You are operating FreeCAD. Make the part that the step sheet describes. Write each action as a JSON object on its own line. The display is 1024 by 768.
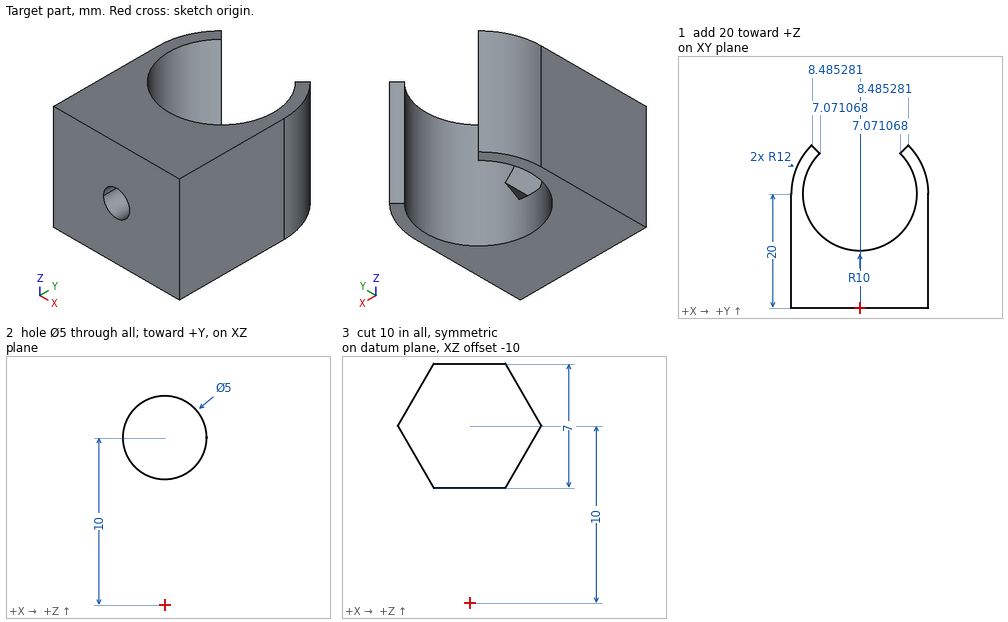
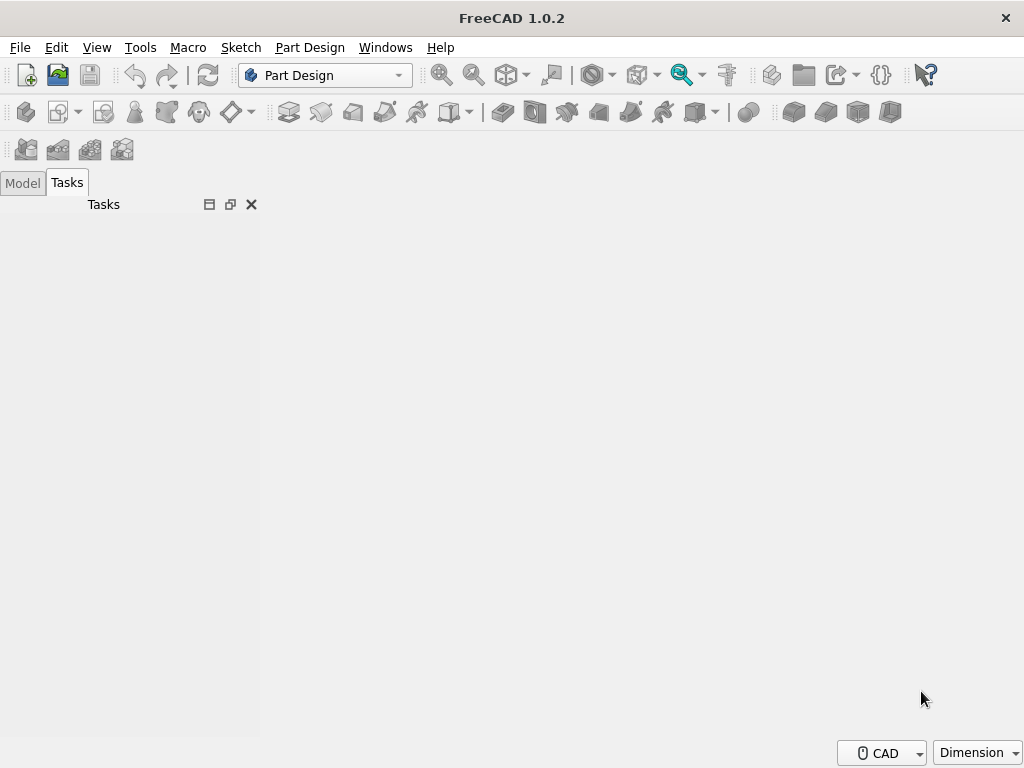
{"action": "left_click", "coordinate": [26, 76]}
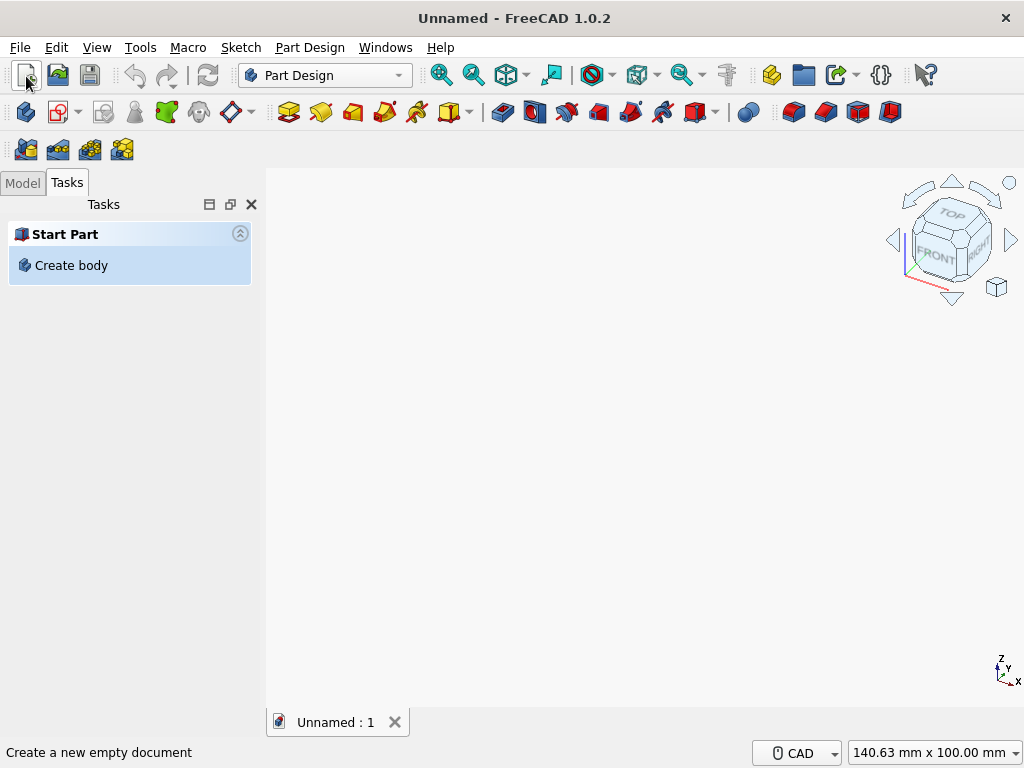
{"action": "left_click", "coordinate": [58, 112]}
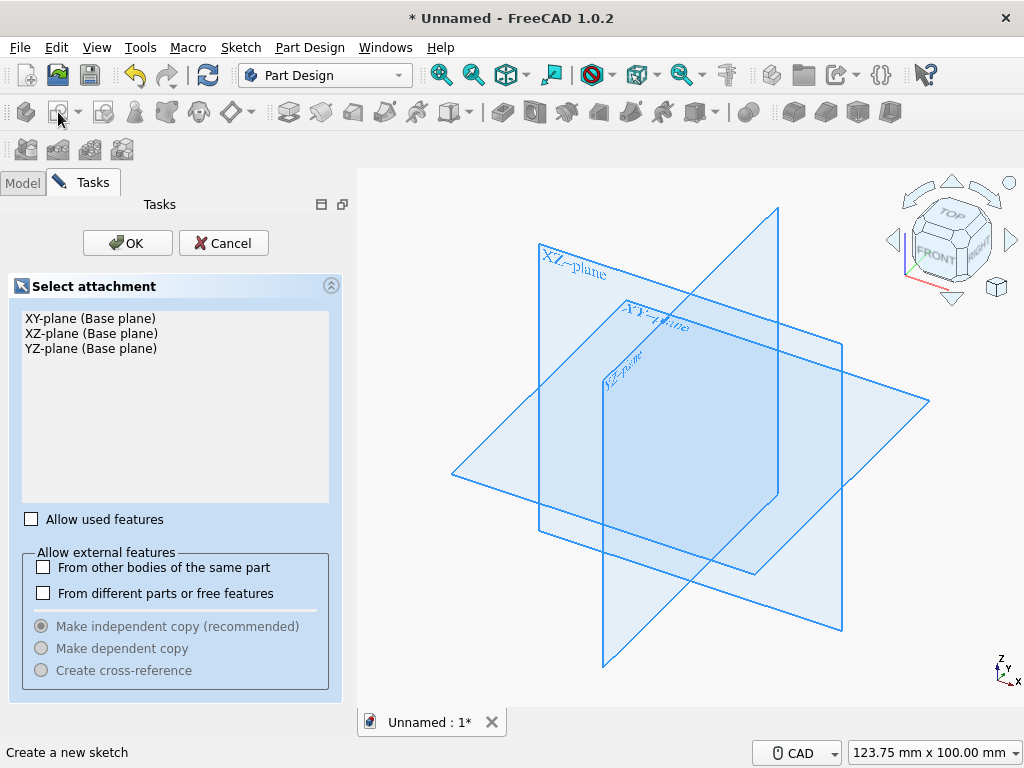
{"action": "left_click", "coordinate": [82, 318]}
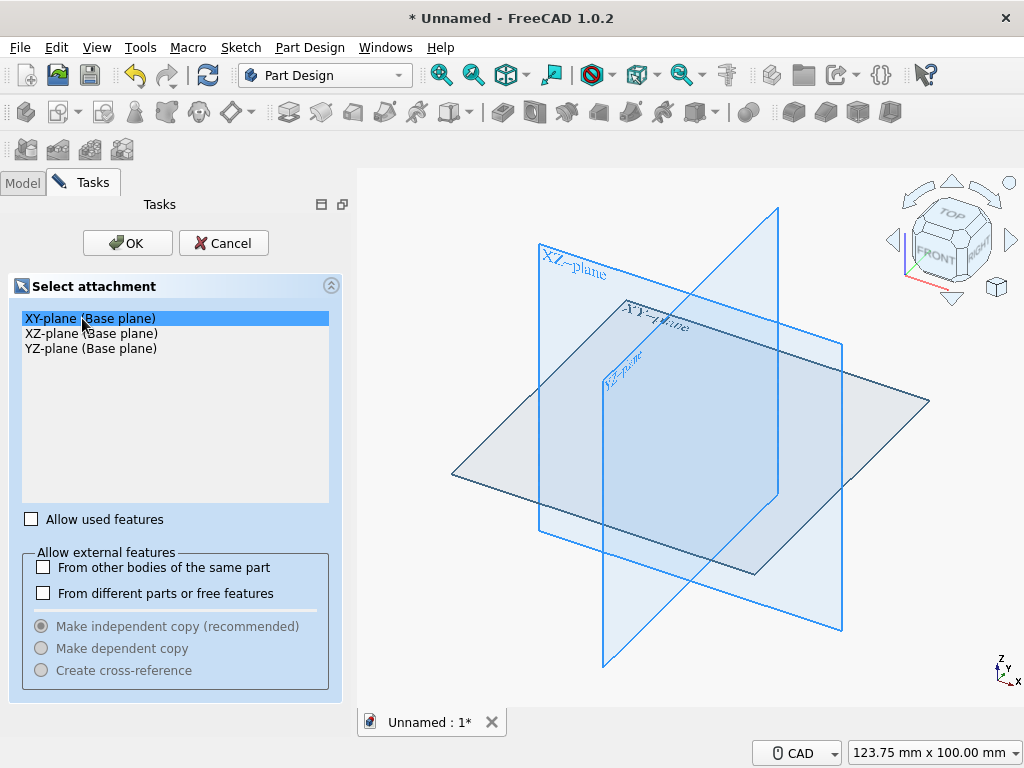
{"action": "left_click", "coordinate": [128, 243]}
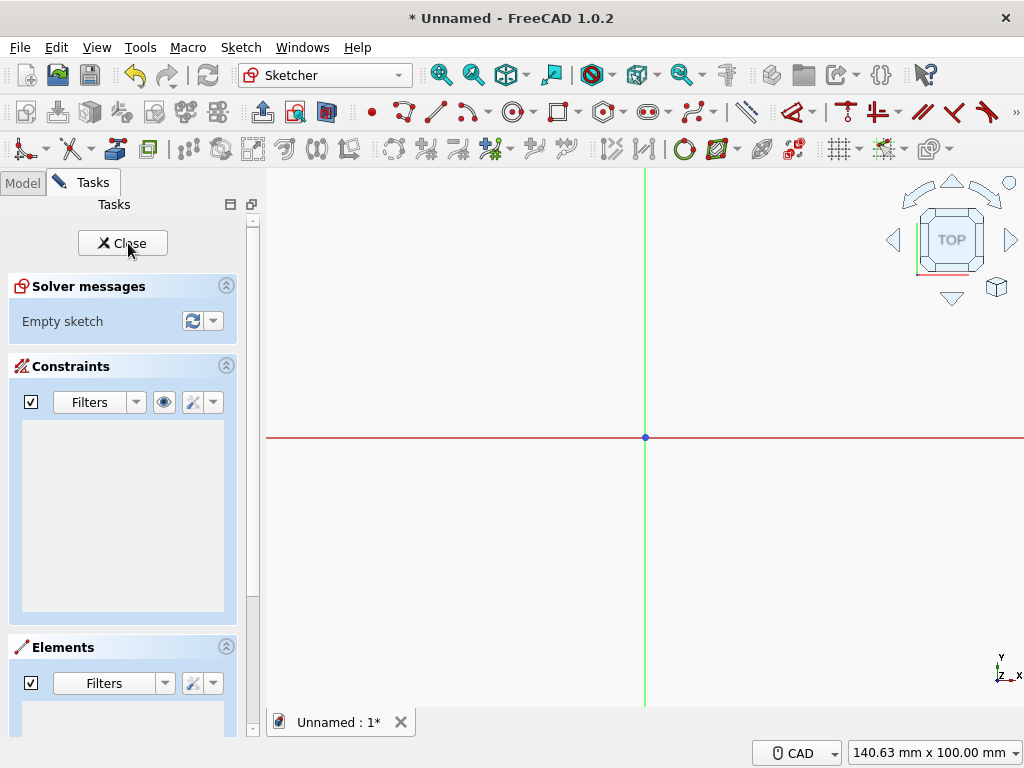
{"action": "scroll", "coordinate": [701, 298], "scroll_direction": "up", "scroll_amount": 4}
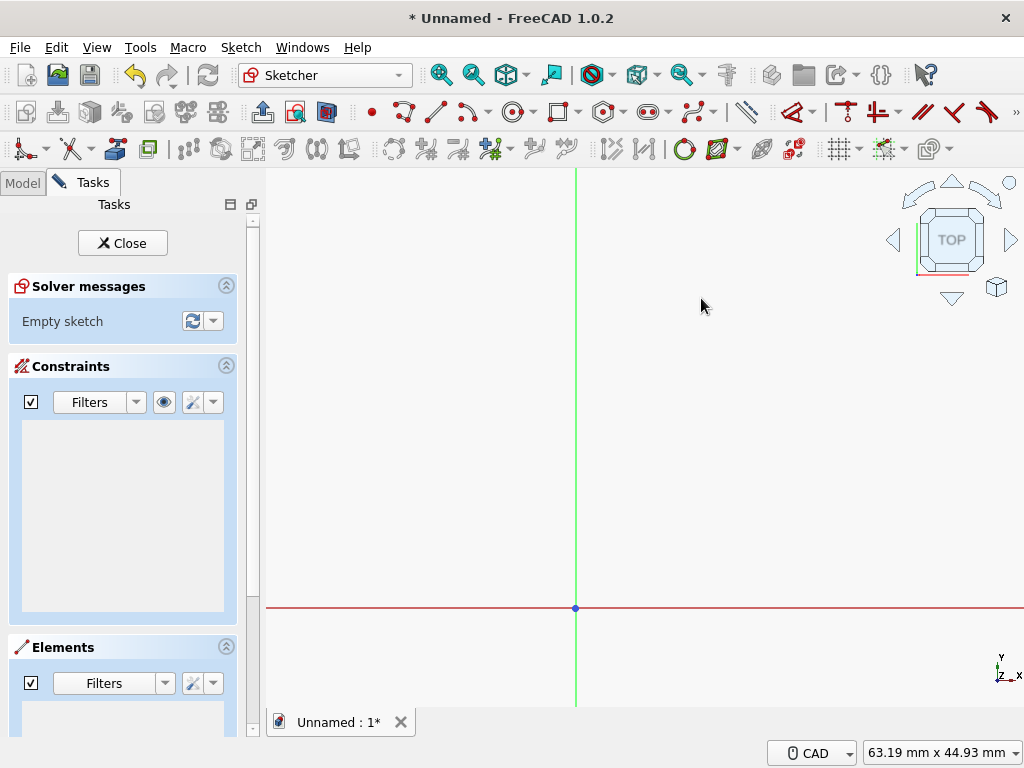
{"action": "key", "text": "g m"}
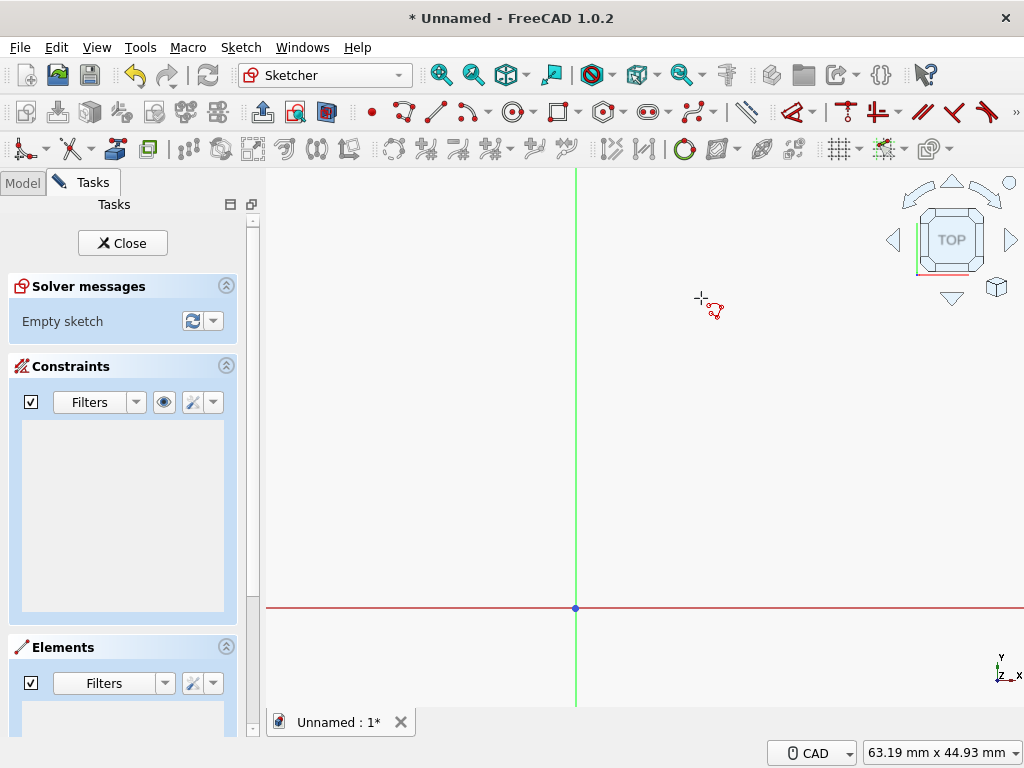
{"action": "left_click", "coordinate": [432, 368]}
{"action": "left_click", "coordinate": [432, 608]}
{"action": "left_click", "coordinate": [720, 599]}
{"action": "left_click", "coordinate": [720, 368]}
{"action": "right_click", "coordinate": [720, 368]}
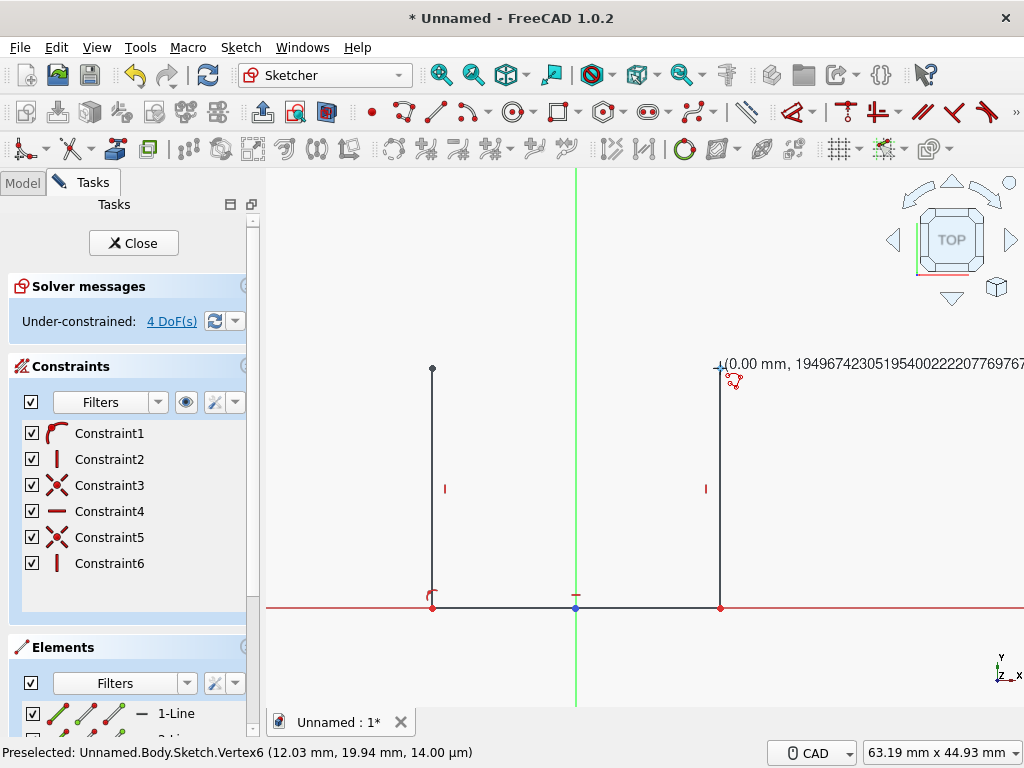
{"action": "left_click", "coordinate": [436, 112]}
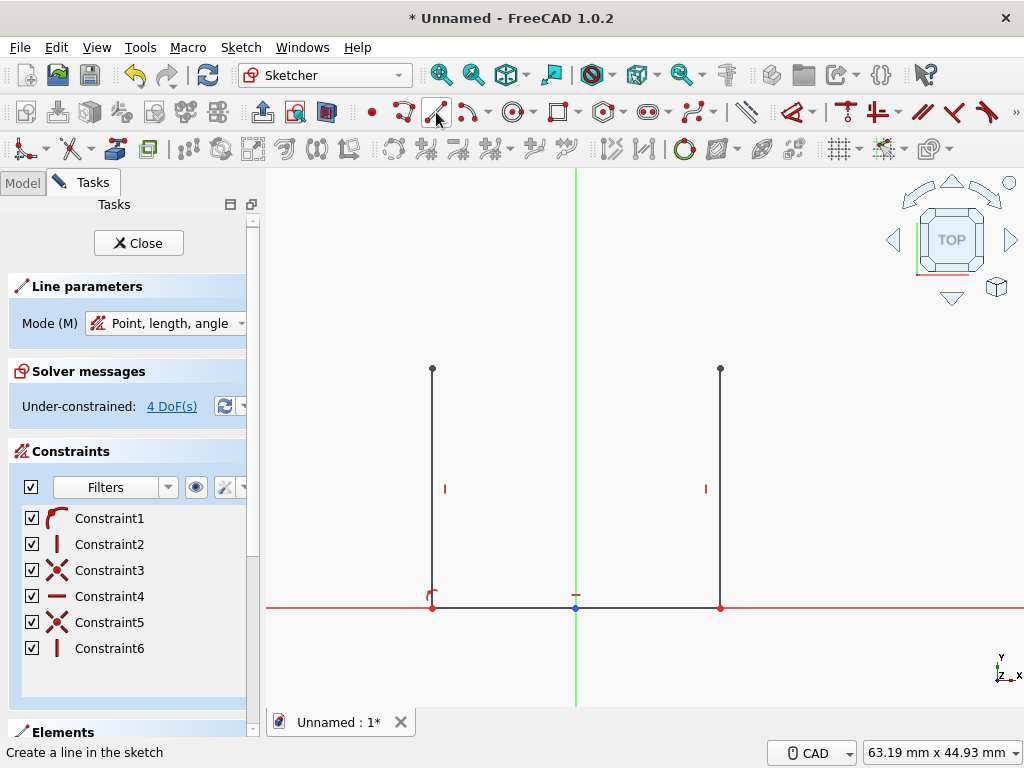
{"action": "left_click", "coordinate": [677, 266]}
{"action": "left_click", "coordinate": [660, 283]}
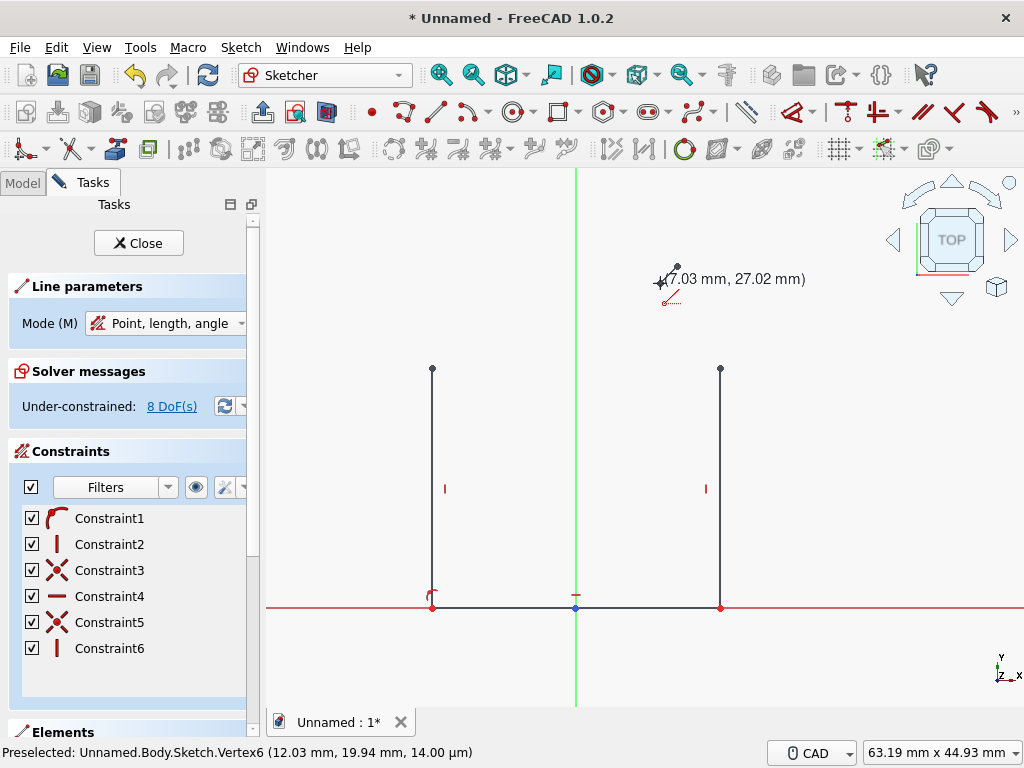
{"action": "left_click", "coordinate": [491, 283]}
{"action": "left_click", "coordinate": [474, 266]}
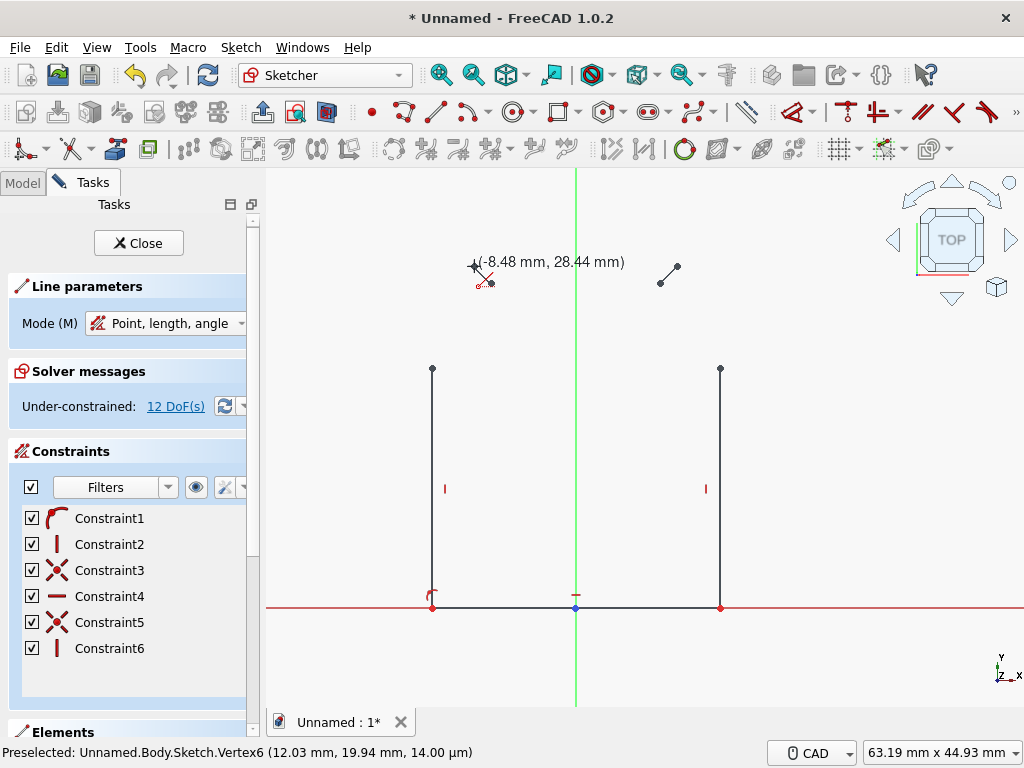
{"action": "left_click", "coordinate": [490, 112]}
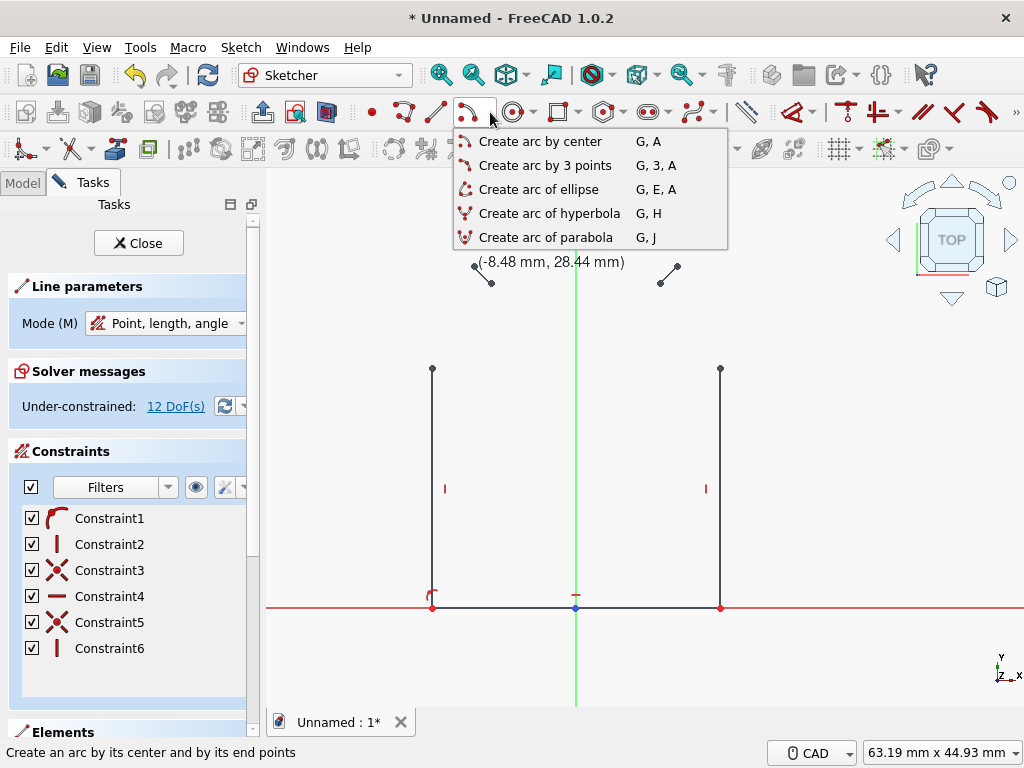
{"action": "left_click", "coordinate": [590, 165]}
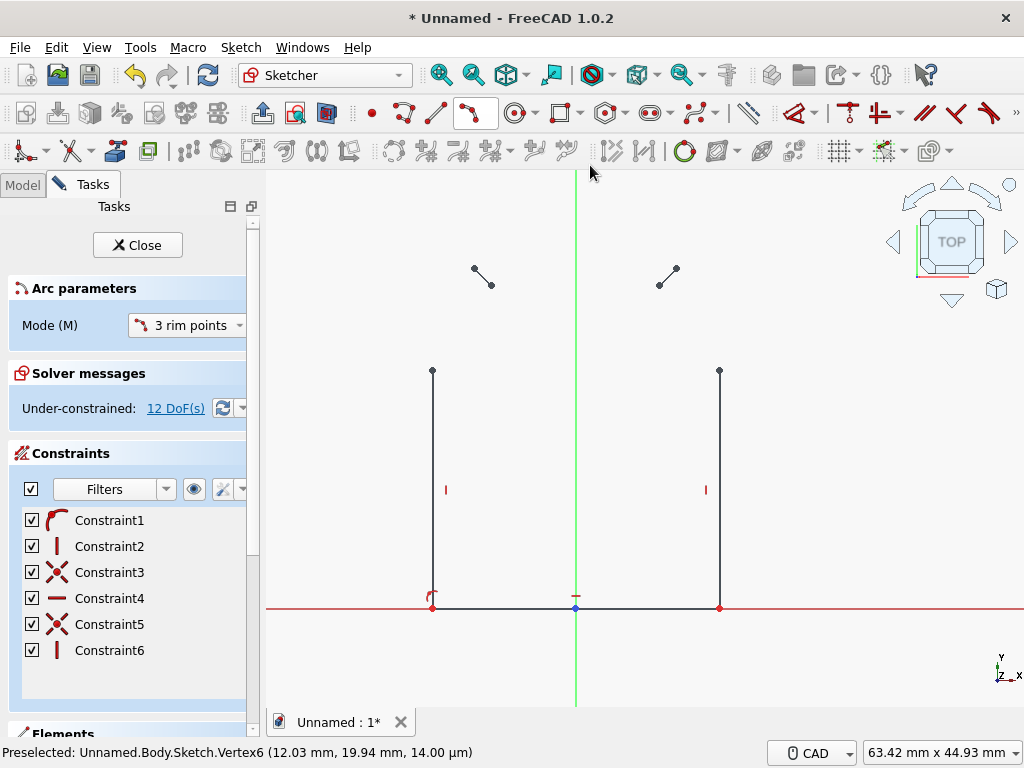
{"action": "left_click", "coordinate": [720, 370]}